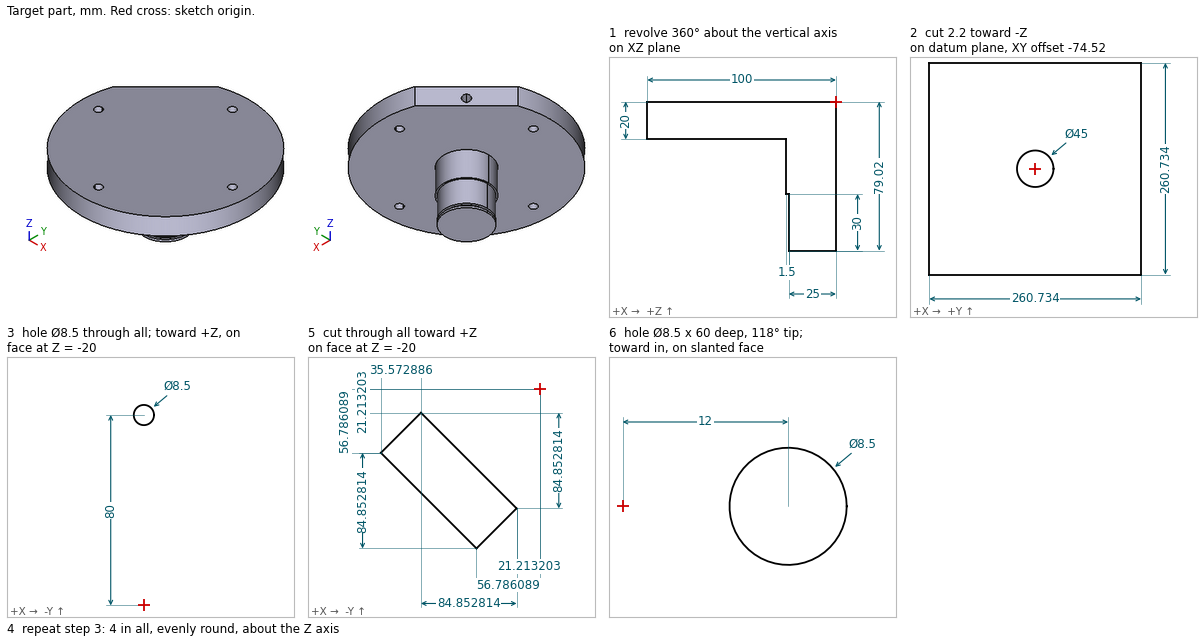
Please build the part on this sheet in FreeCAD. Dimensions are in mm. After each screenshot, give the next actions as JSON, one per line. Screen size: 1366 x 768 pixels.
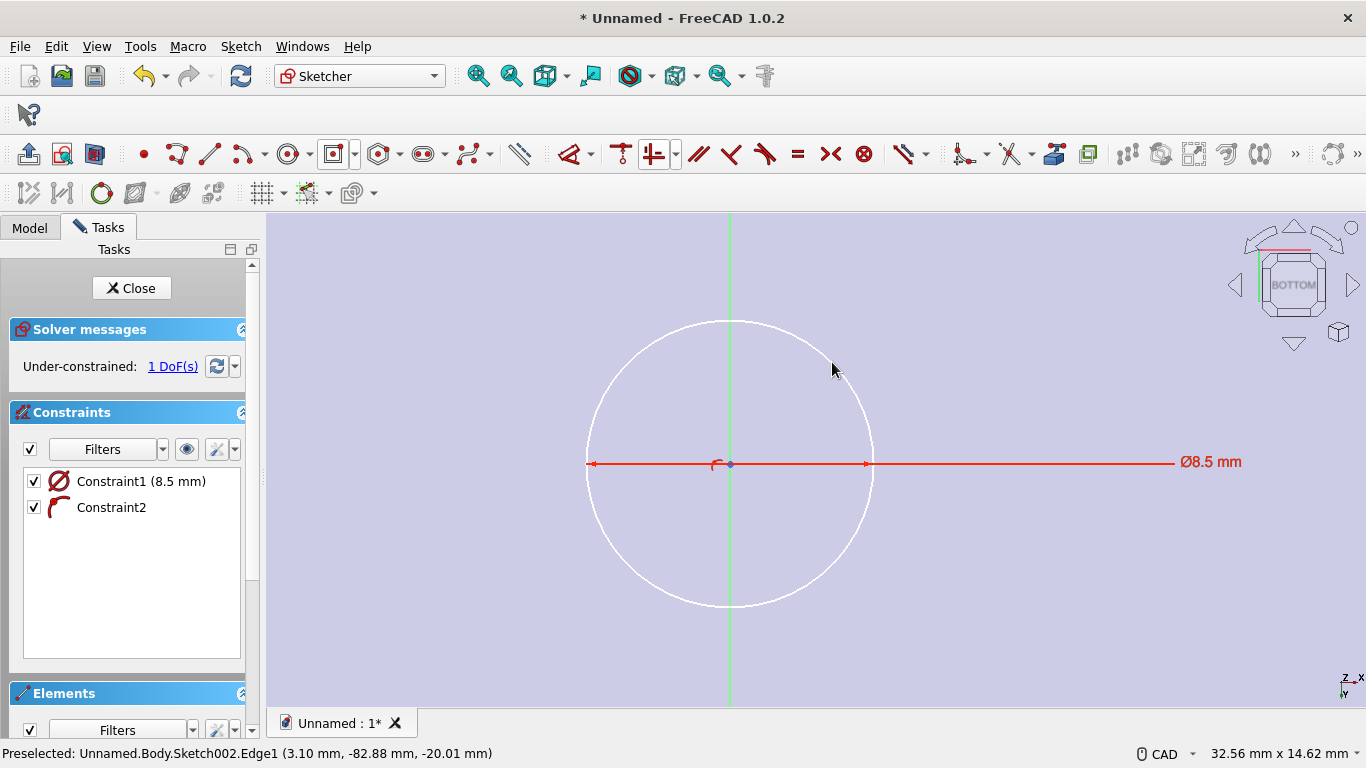
{"action": "key", "text": "d"}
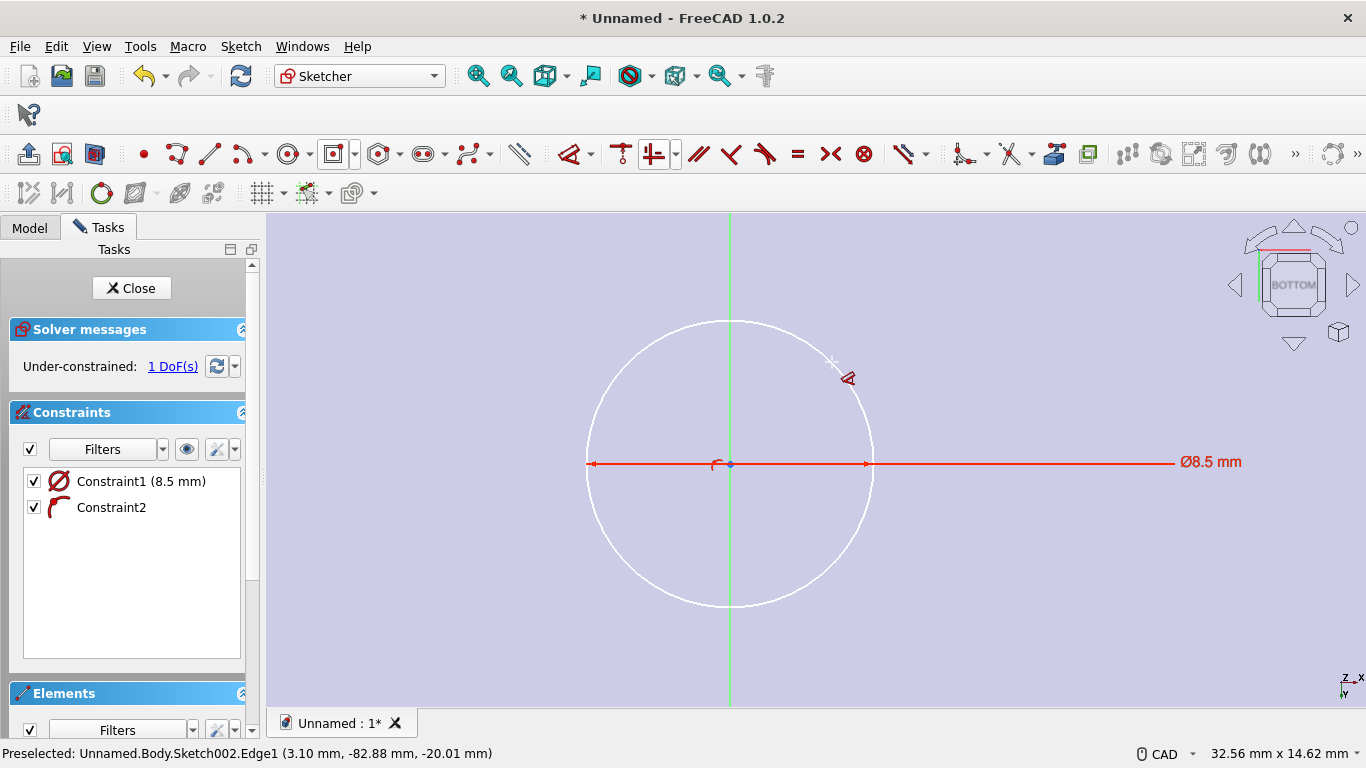
{"action": "left_click", "coordinate": [730, 464]}
{"action": "left_click", "coordinate": [764, 572]}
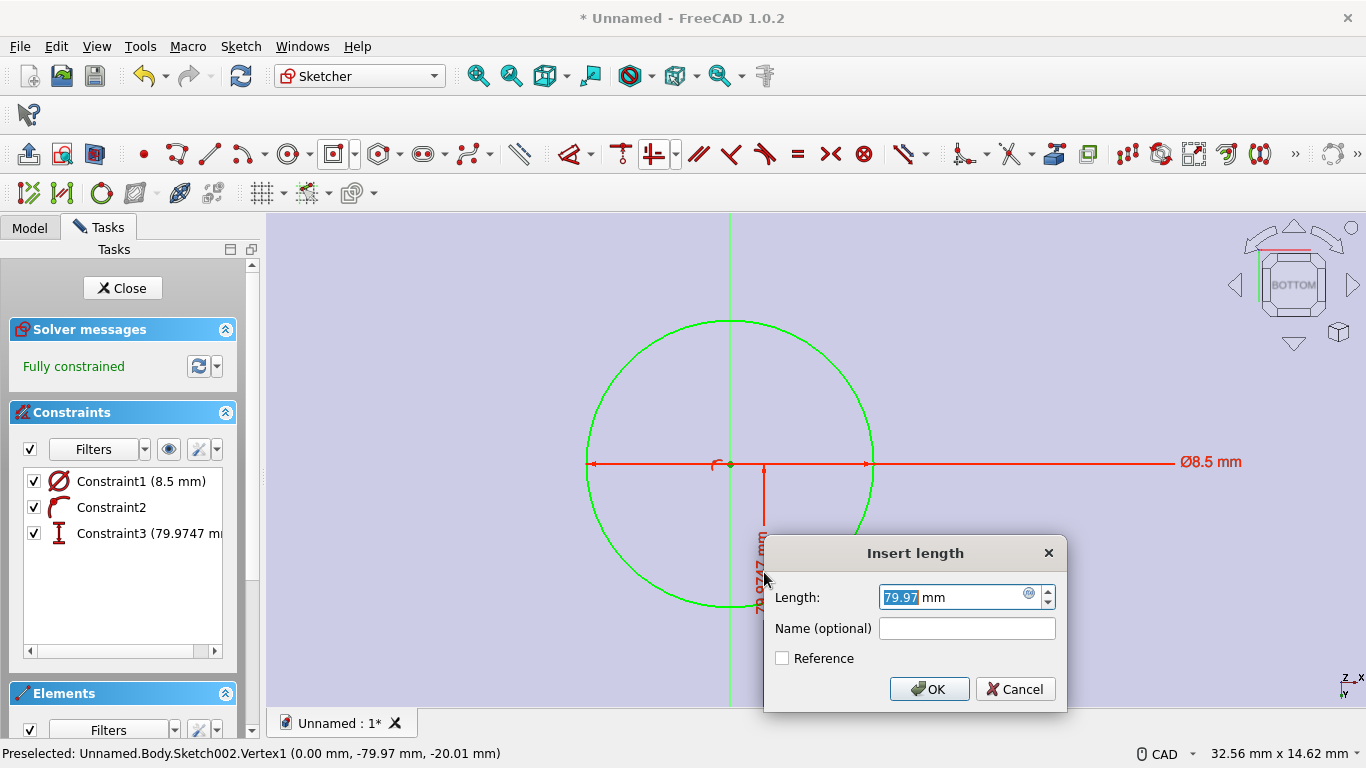
{"action": "type", "text": "80"}
{"action": "key", "text": "Return"}
{"action": "key", "text": "Escape"}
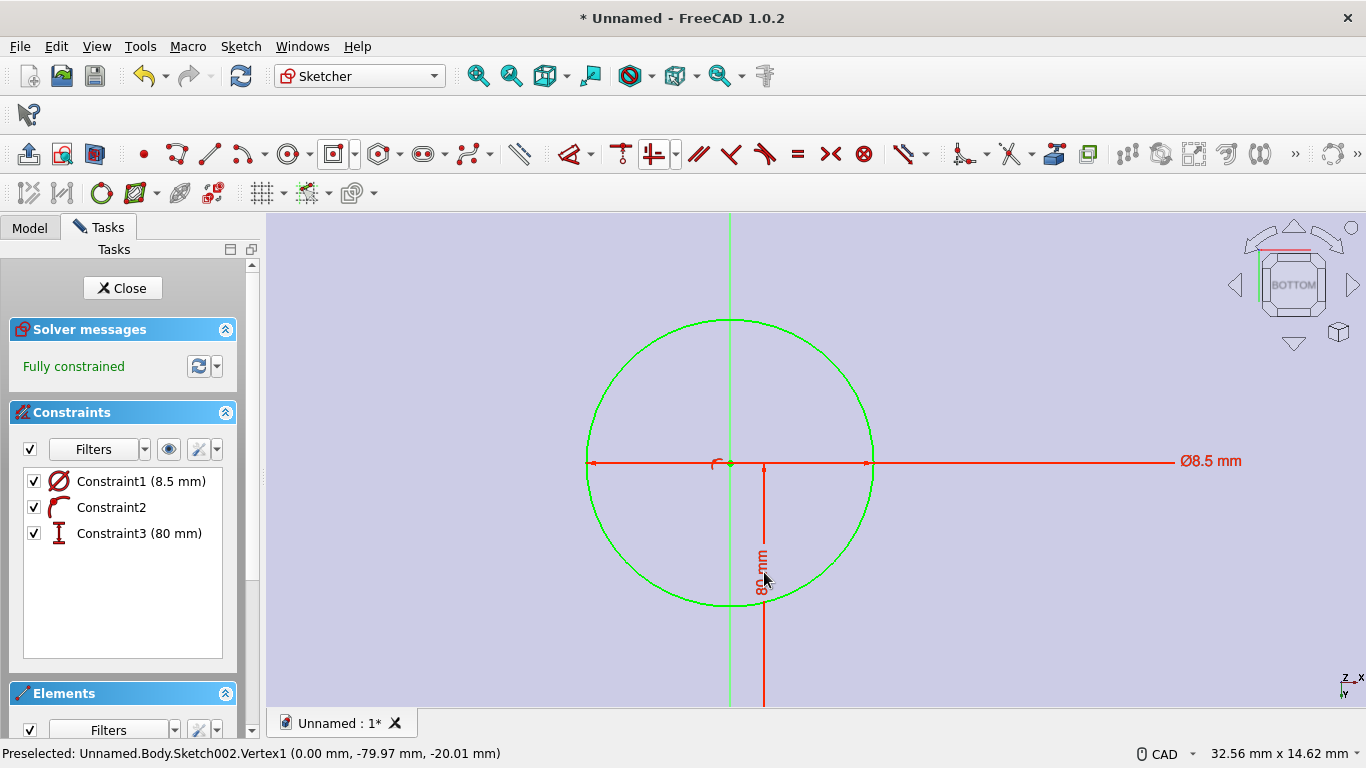
{"action": "left_click", "coordinate": [123, 288]}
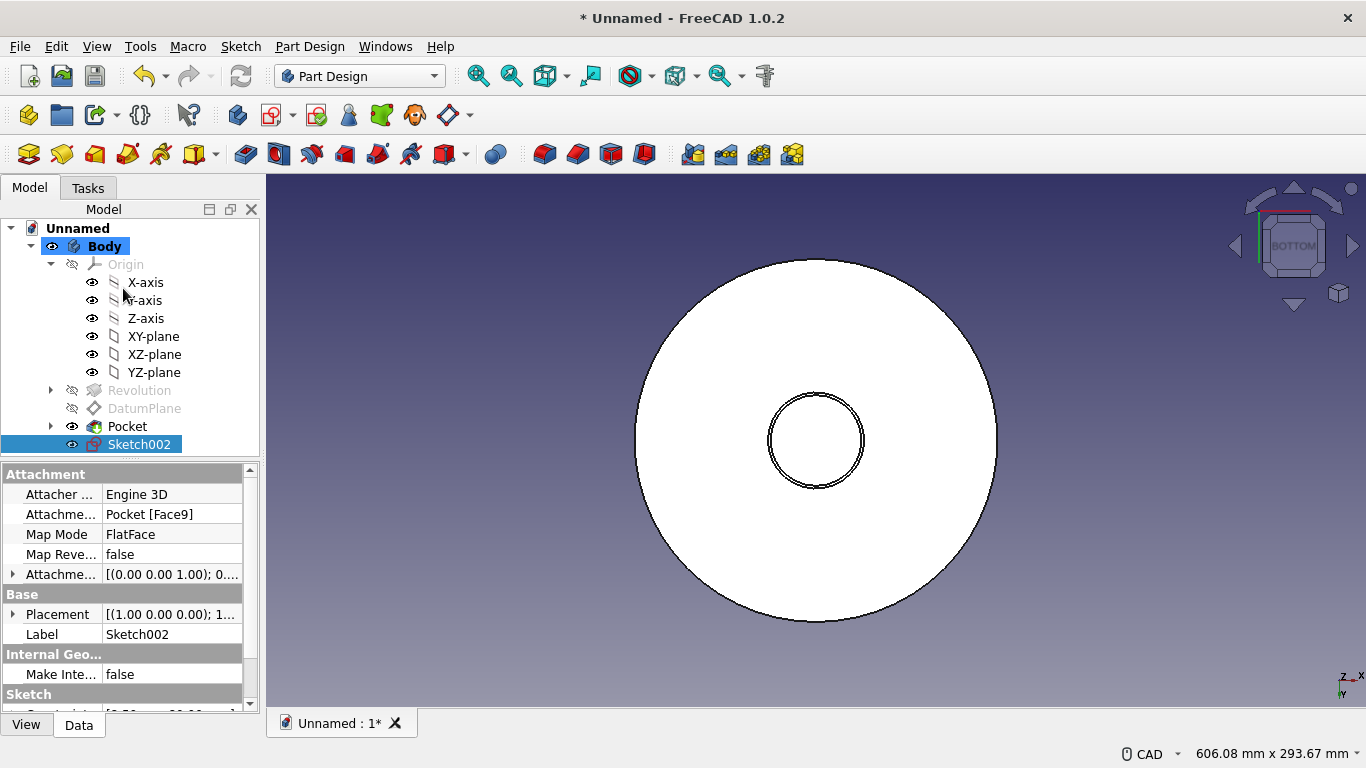
{"action": "left_click", "coordinate": [279, 154]}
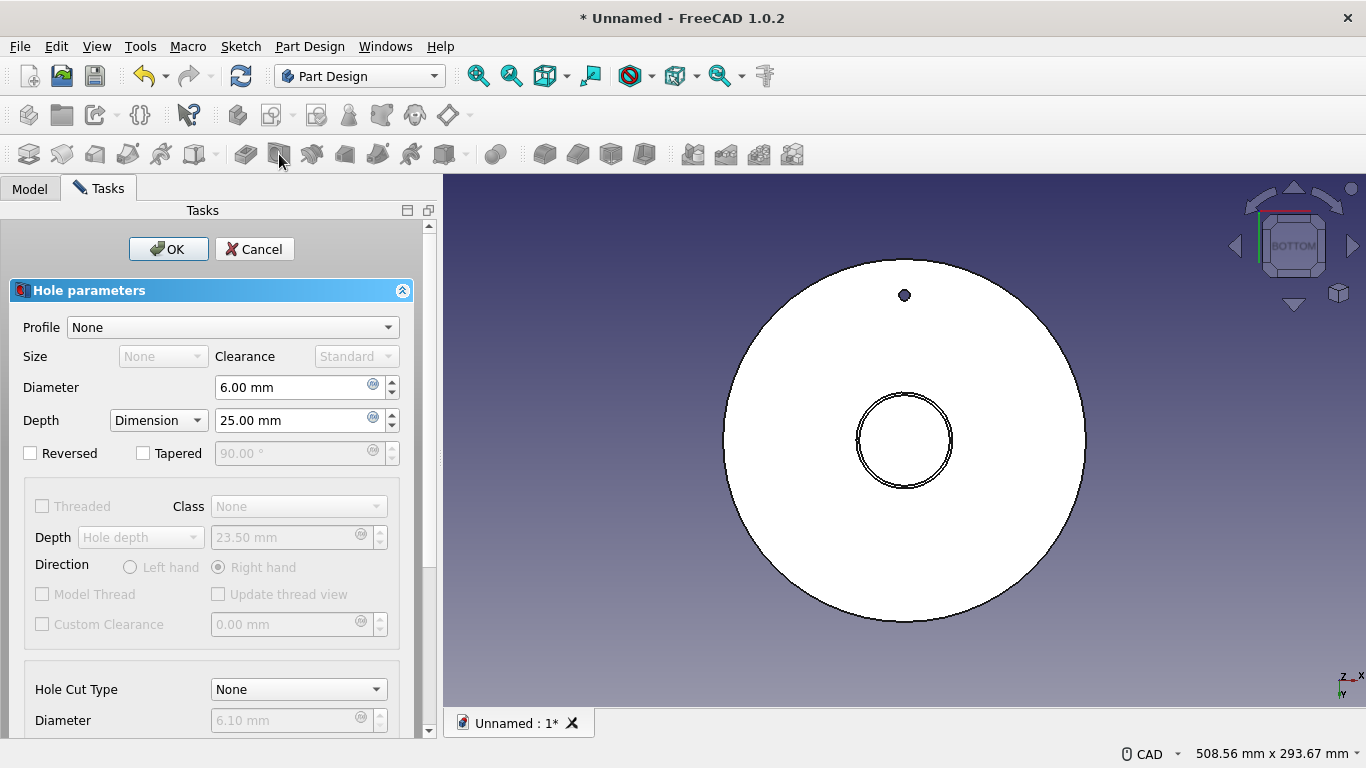
{"action": "triple_click", "coordinate": [300, 388]}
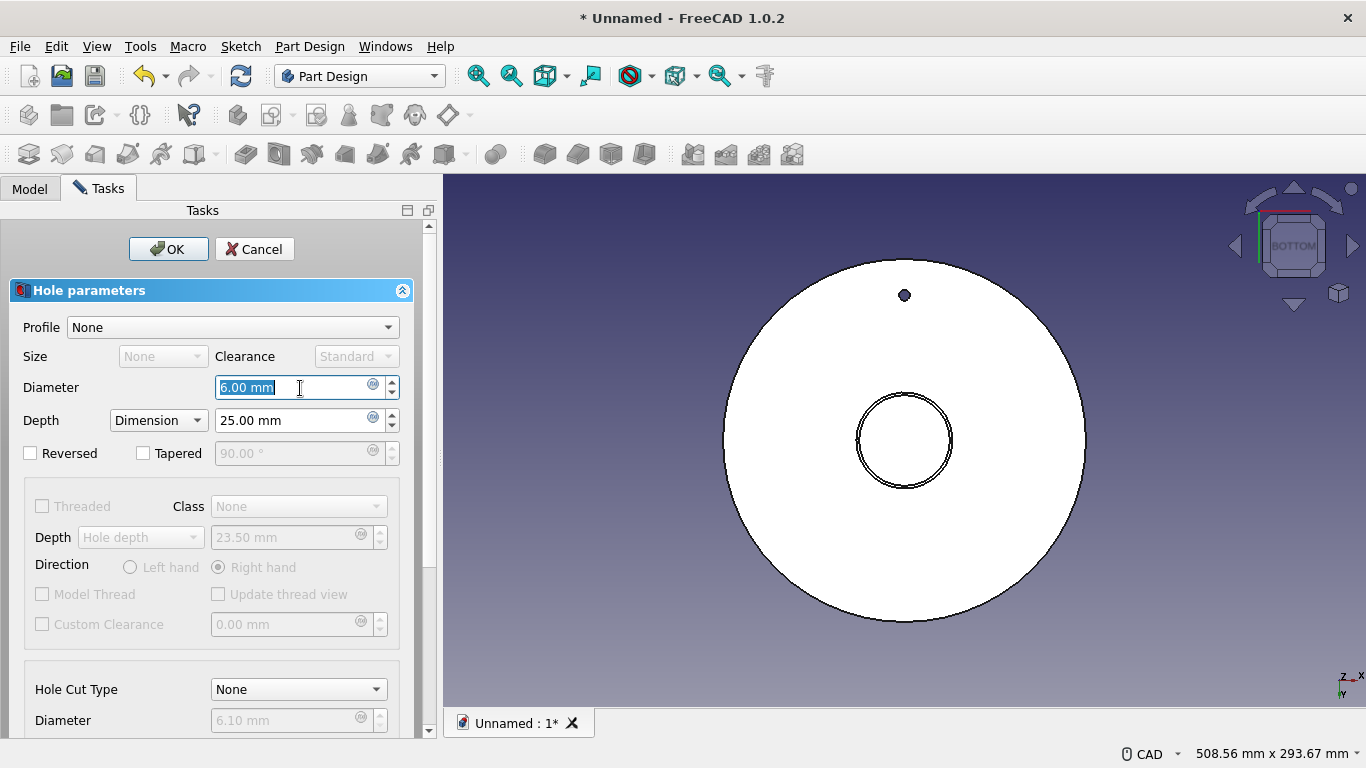
{"action": "type", "text": "8.5"}
{"action": "key", "text": "Tab"}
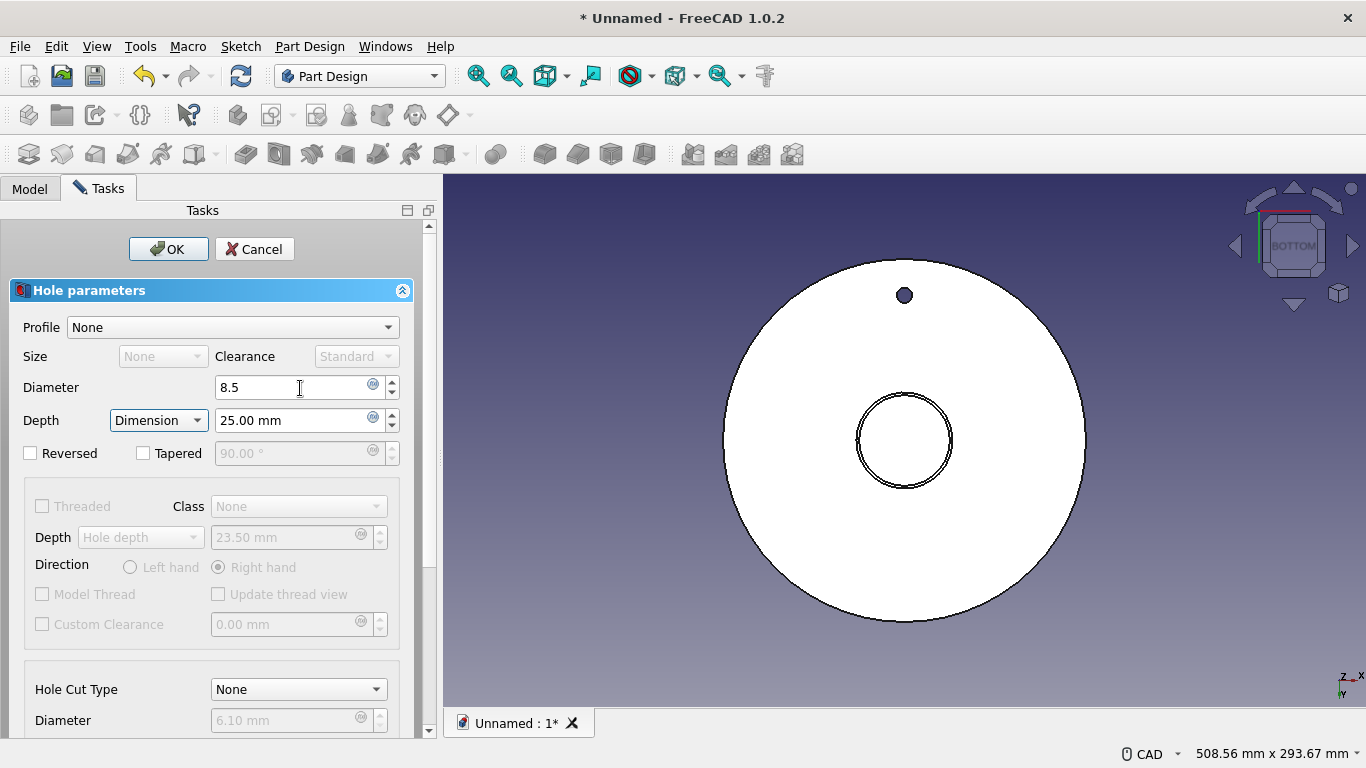
{"action": "left_click", "coordinate": [160, 420]}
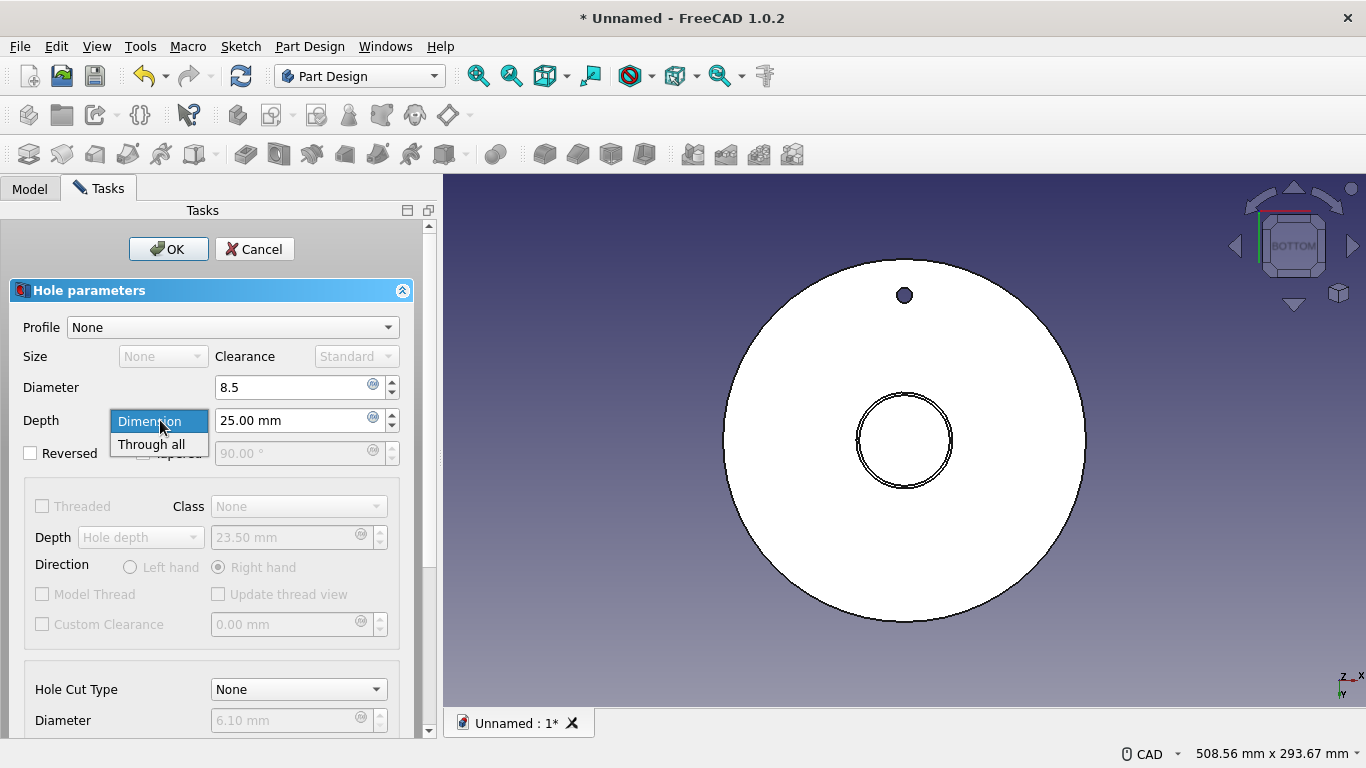
{"action": "left_click", "coordinate": [158, 444]}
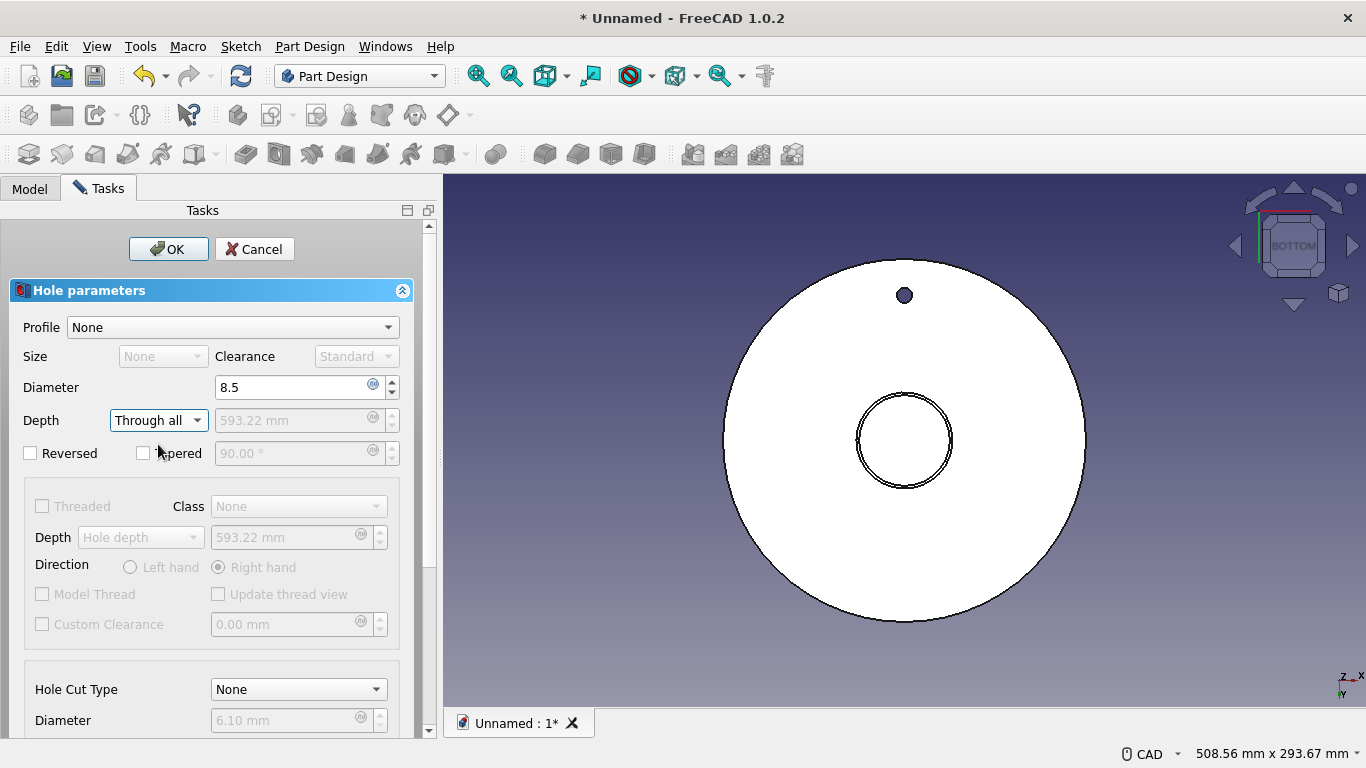
{"action": "left_click", "coordinate": [169, 249]}